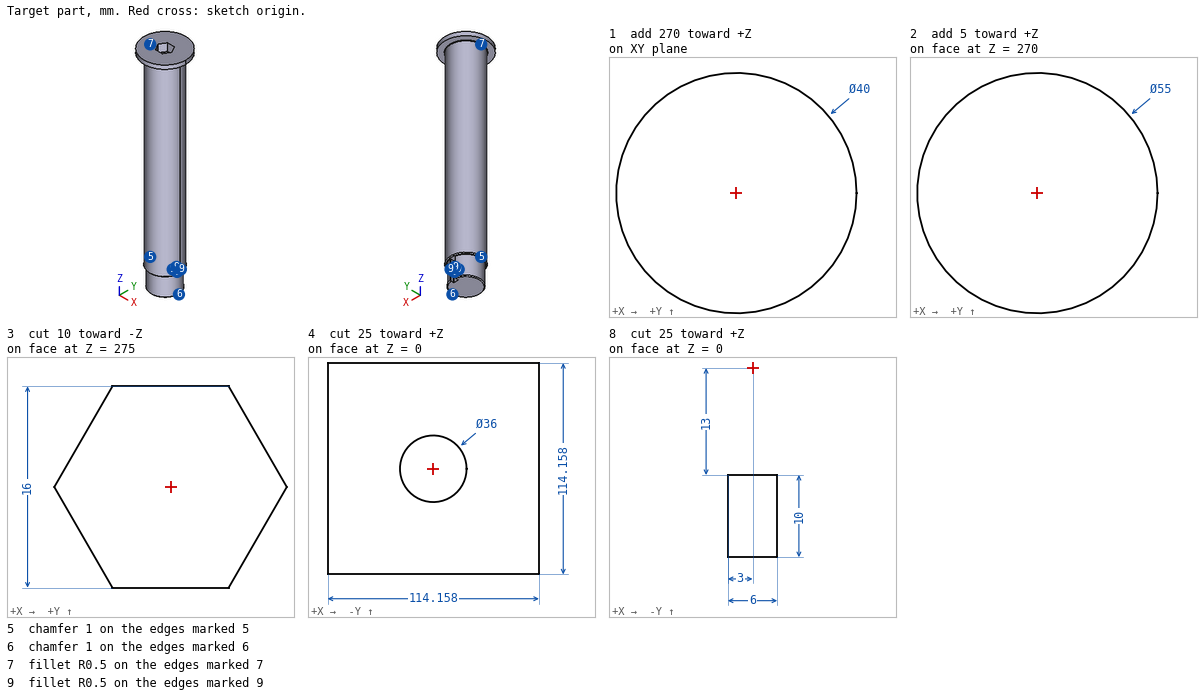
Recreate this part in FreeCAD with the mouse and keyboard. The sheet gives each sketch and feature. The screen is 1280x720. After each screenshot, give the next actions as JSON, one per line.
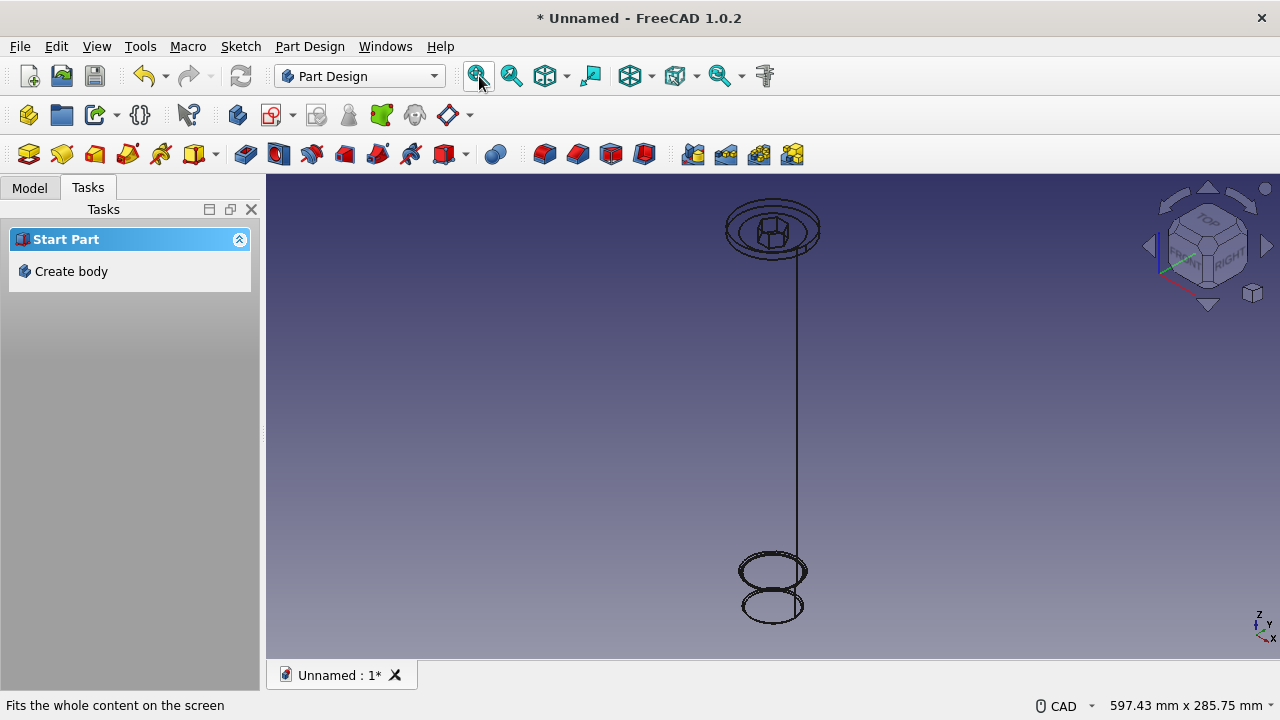
{"action": "left_click", "coordinate": [749, 218]}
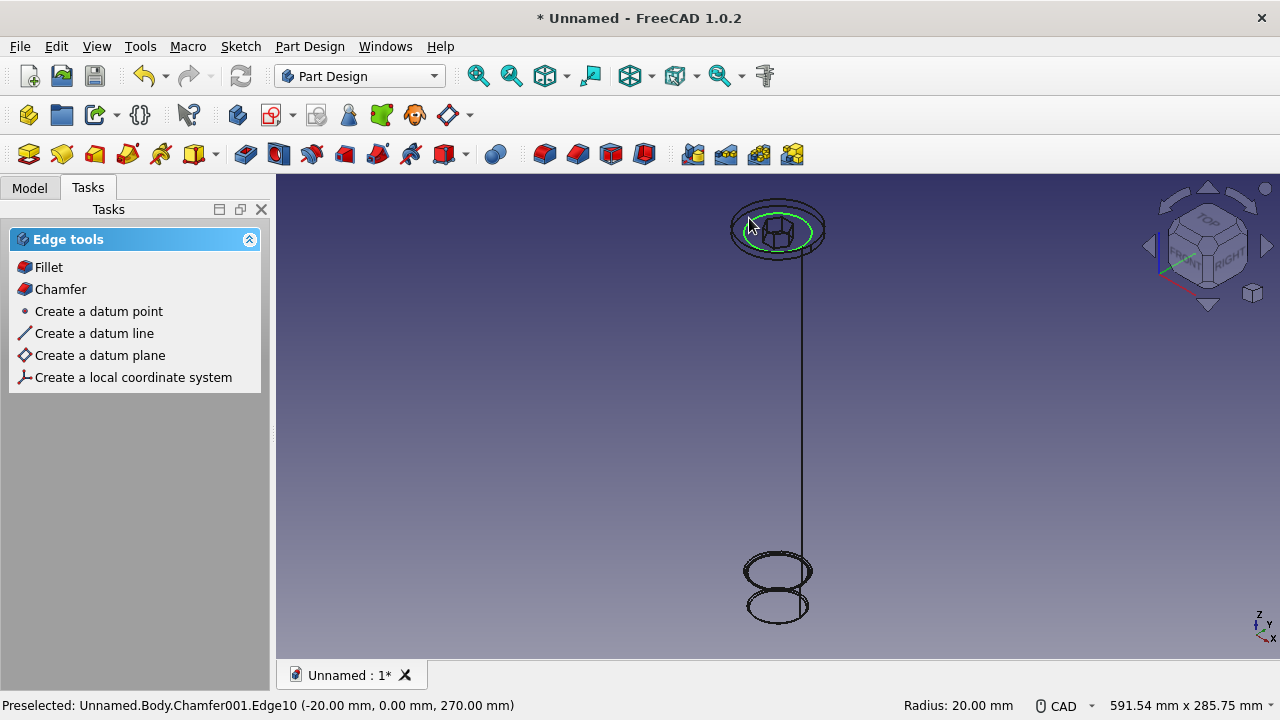
{"action": "key", "text": "v 1"}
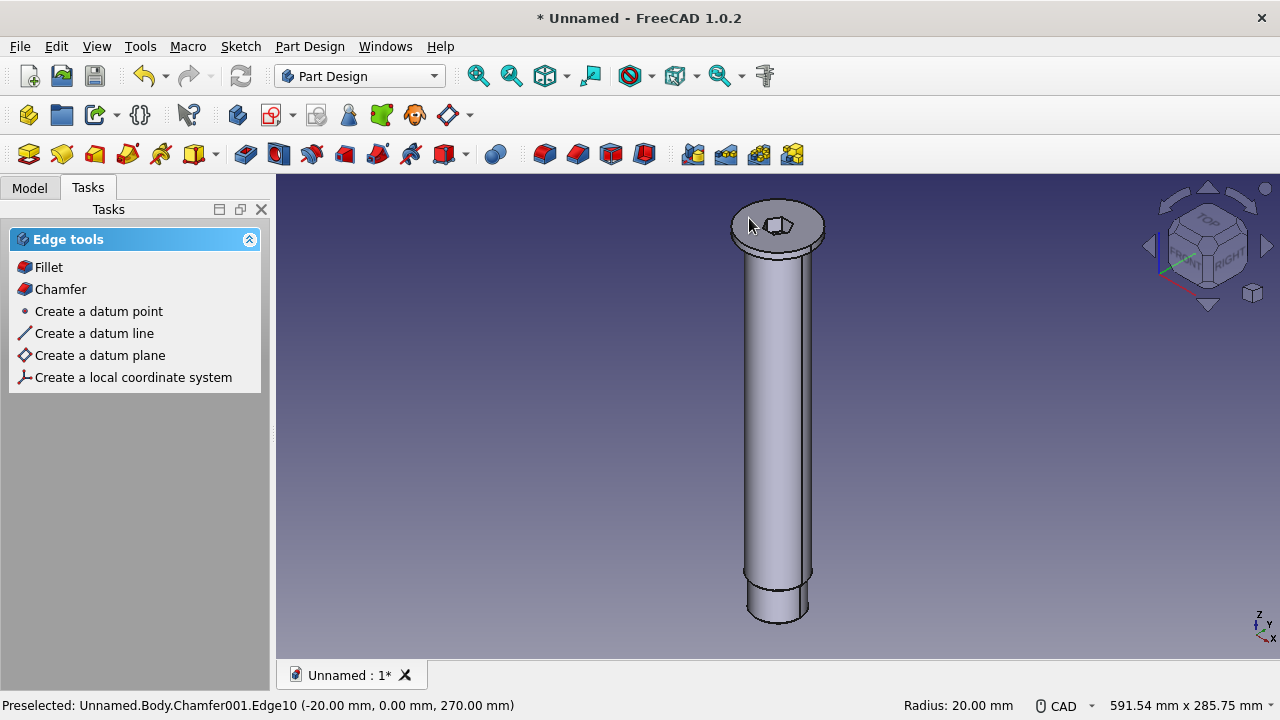
{"action": "left_click", "coordinate": [545, 154]}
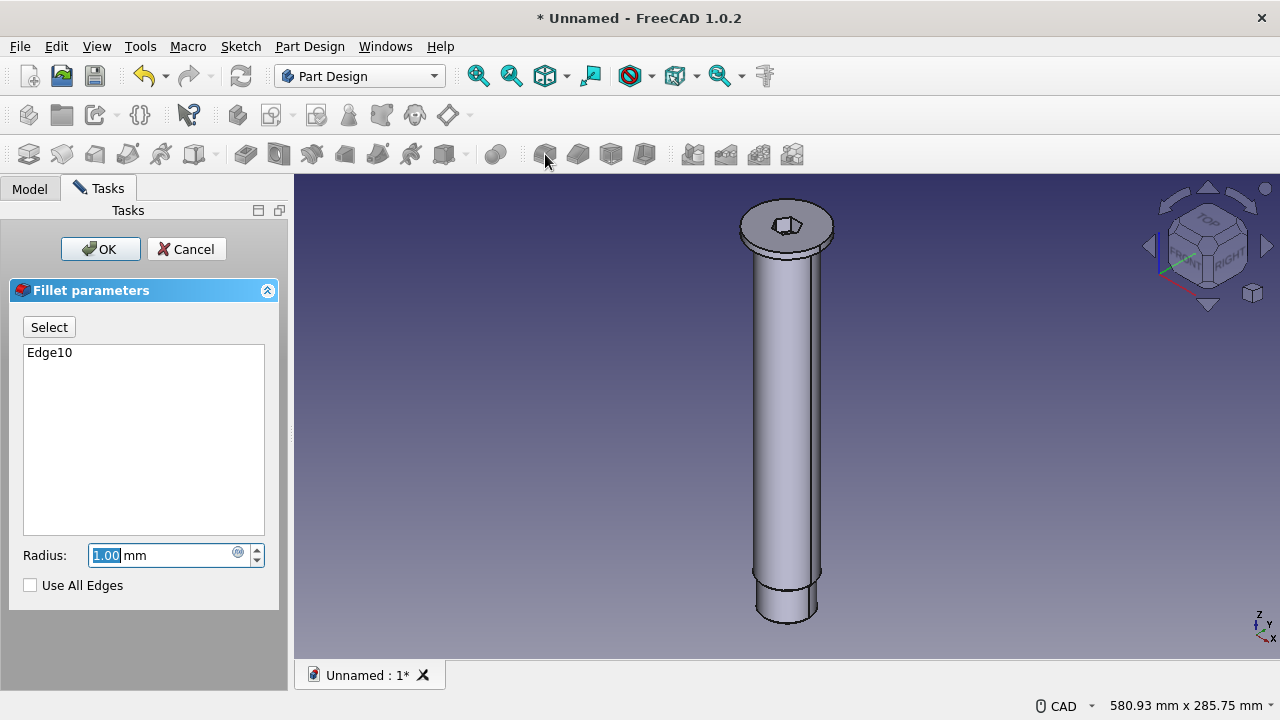
{"action": "type", "text": "0.5"}
{"action": "key", "text": "Tab"}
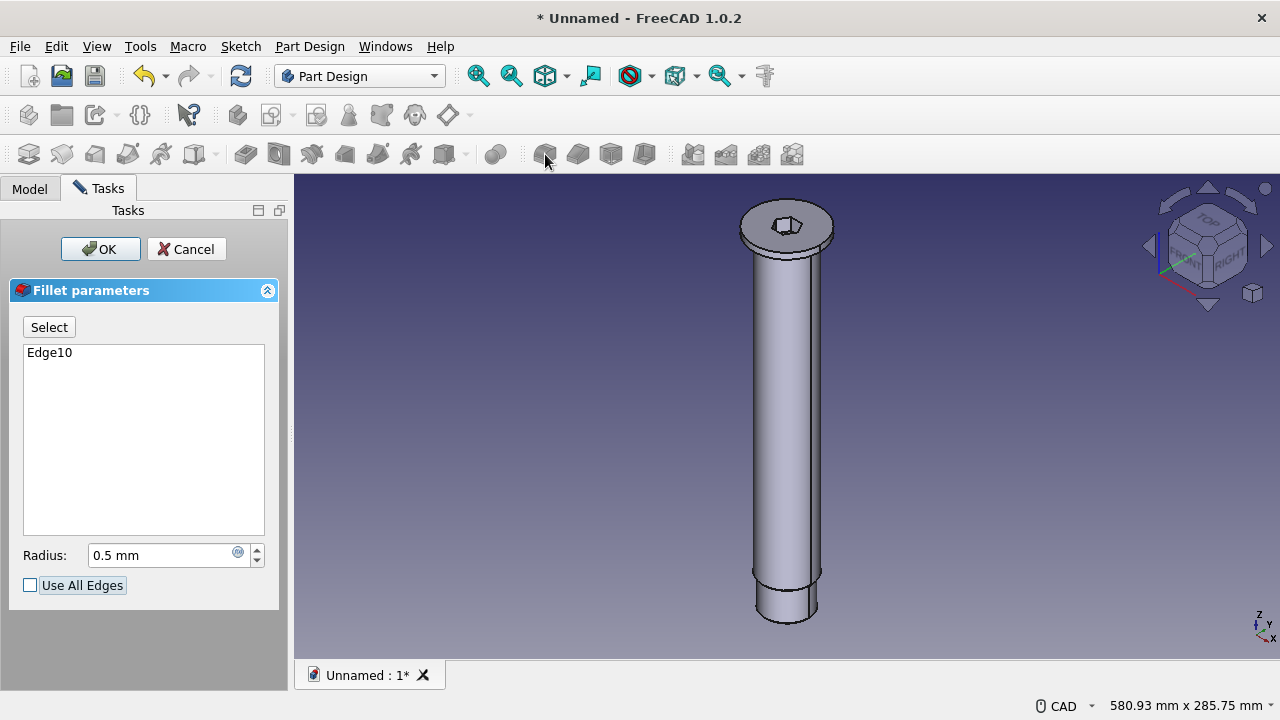
{"action": "left_click", "coordinate": [101, 249]}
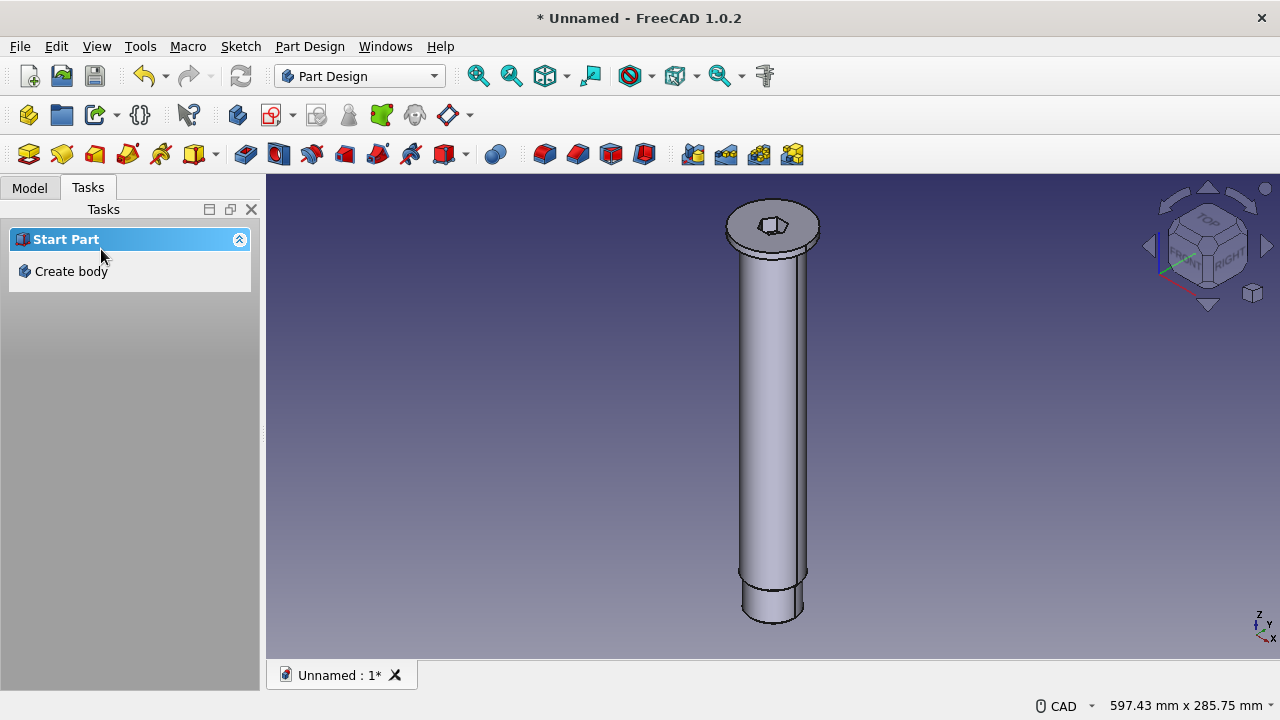
{"action": "key", "text": "5"}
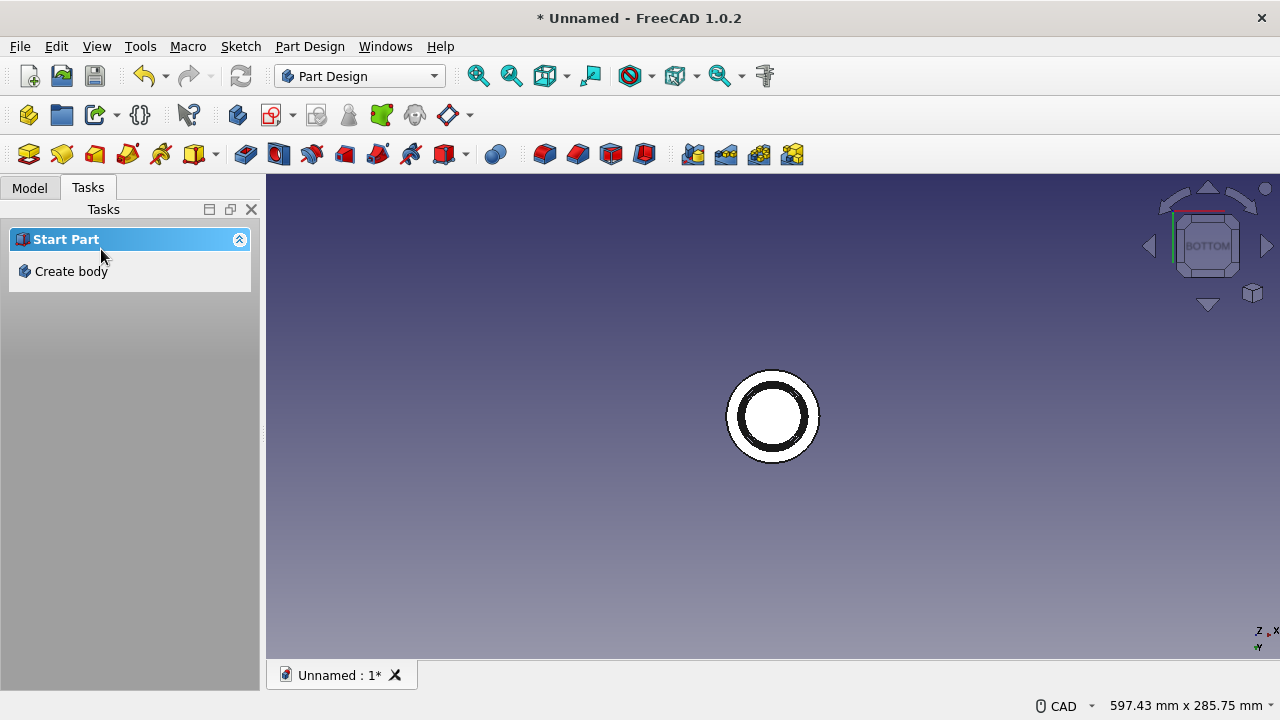
{"action": "left_click", "coordinate": [479, 76]}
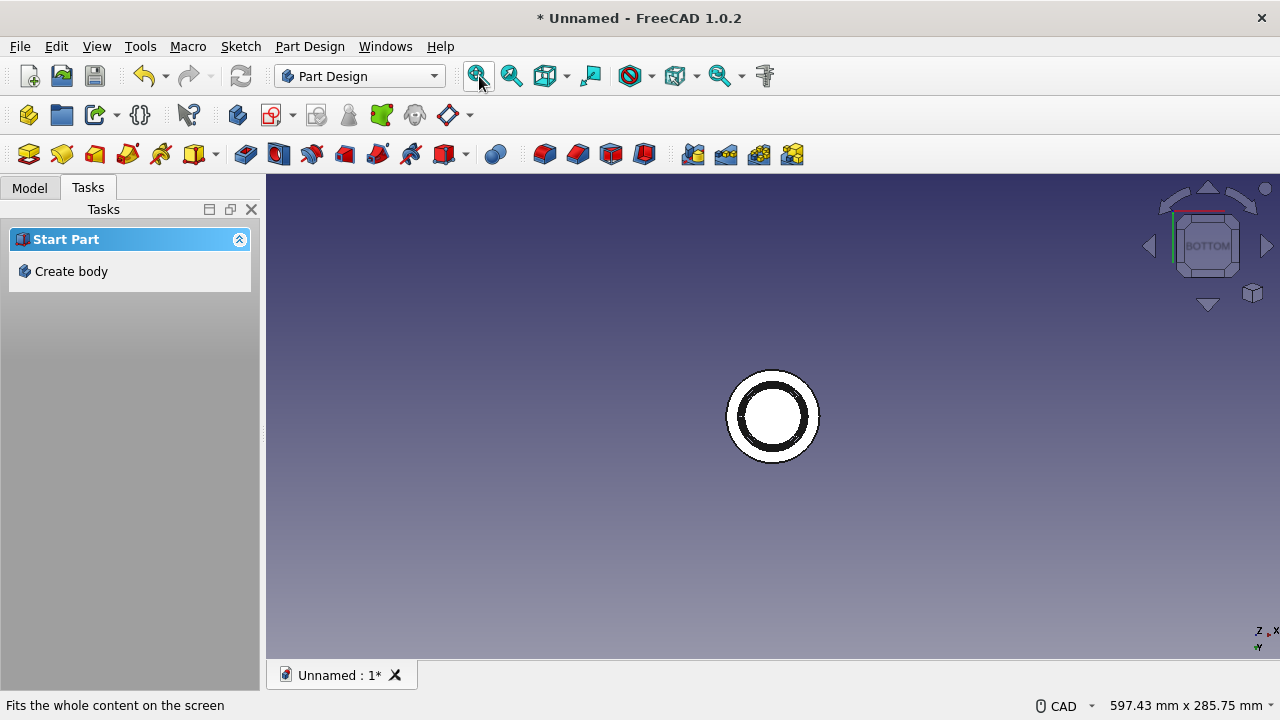
{"action": "left_click", "coordinate": [773, 415]}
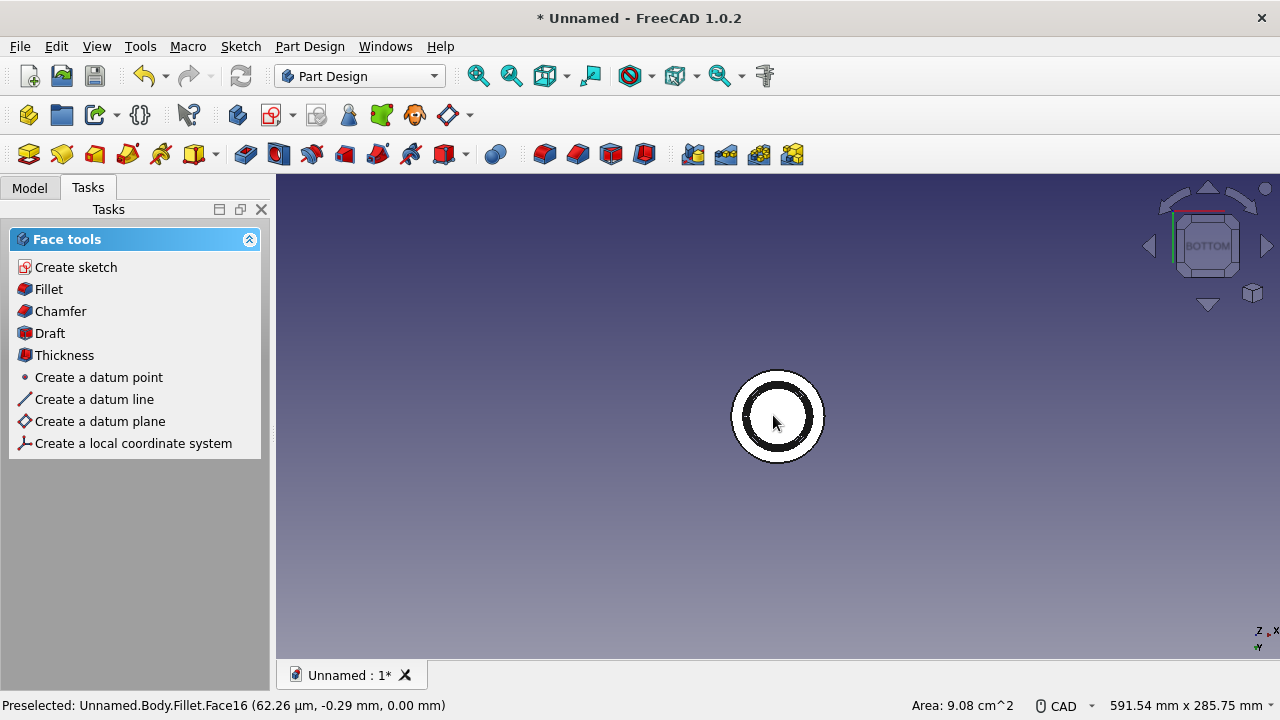
{"action": "left_click", "coordinate": [270, 116]}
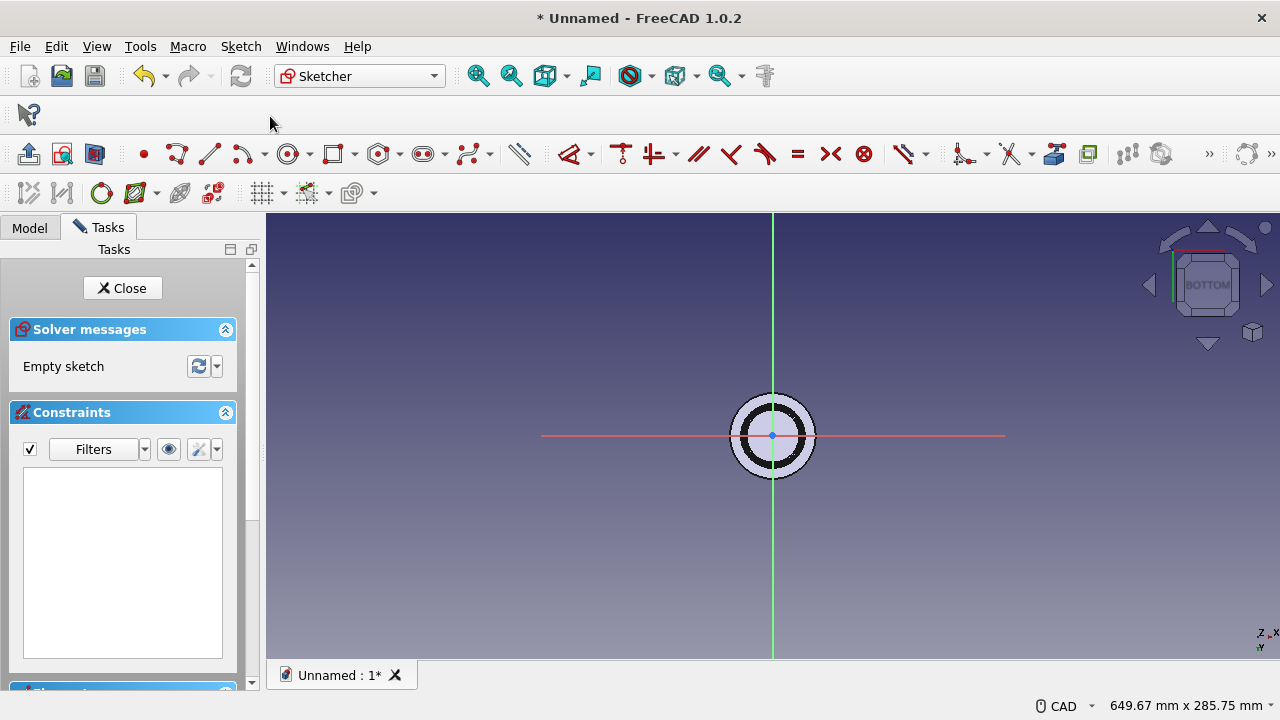
{"action": "scroll", "coordinate": [784, 457], "scroll_direction": "up", "scroll_amount": 10}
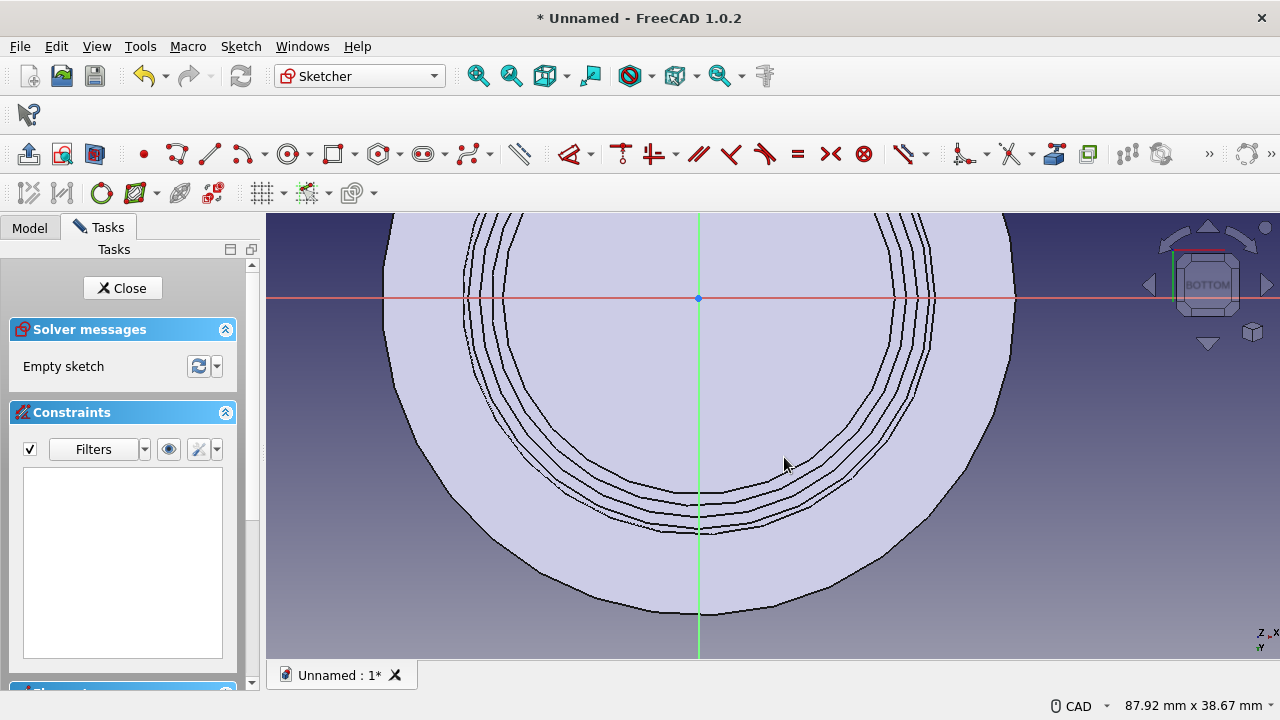
{"action": "left_click", "coordinate": [332, 154]}